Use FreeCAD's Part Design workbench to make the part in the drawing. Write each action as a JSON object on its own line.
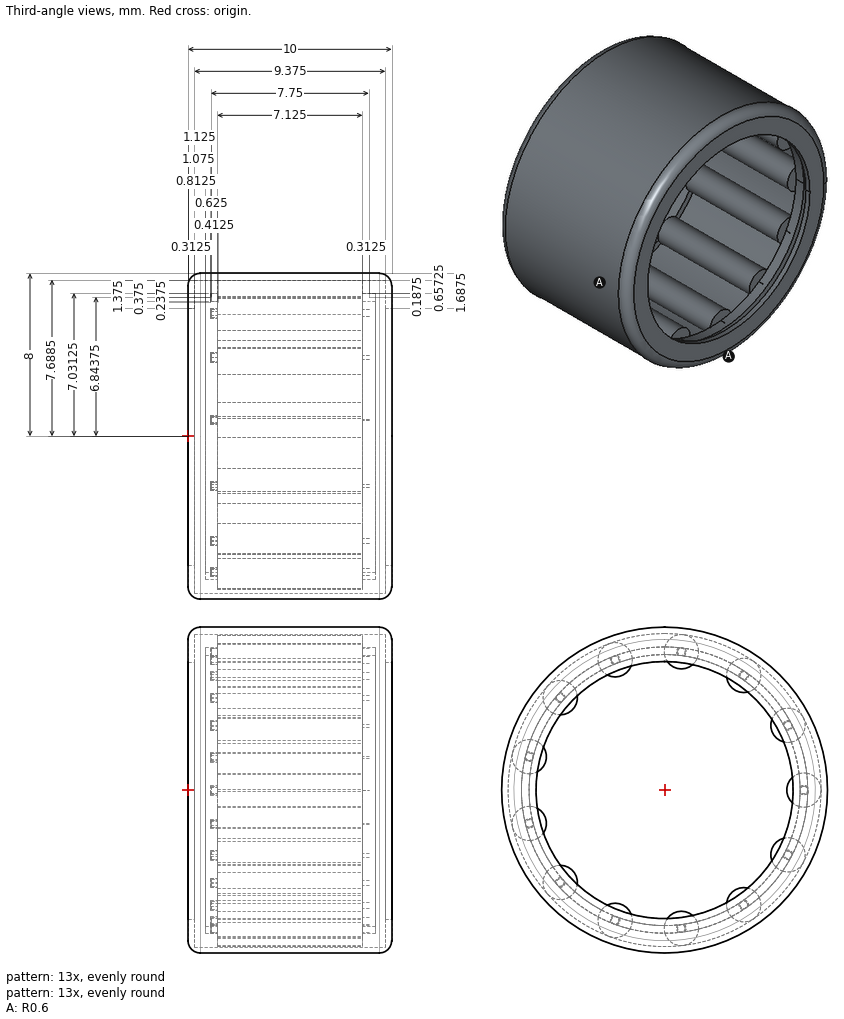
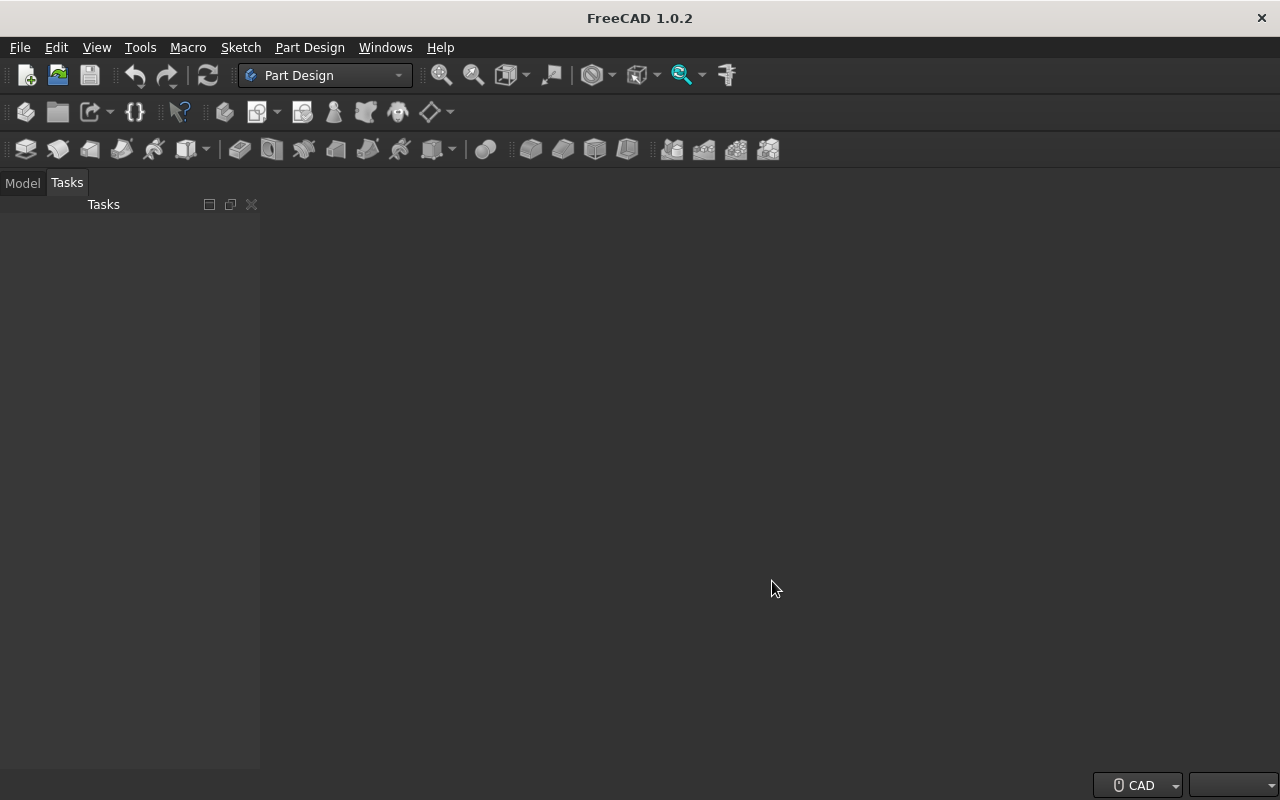
{"action": "left_click", "coordinate": [26, 76]}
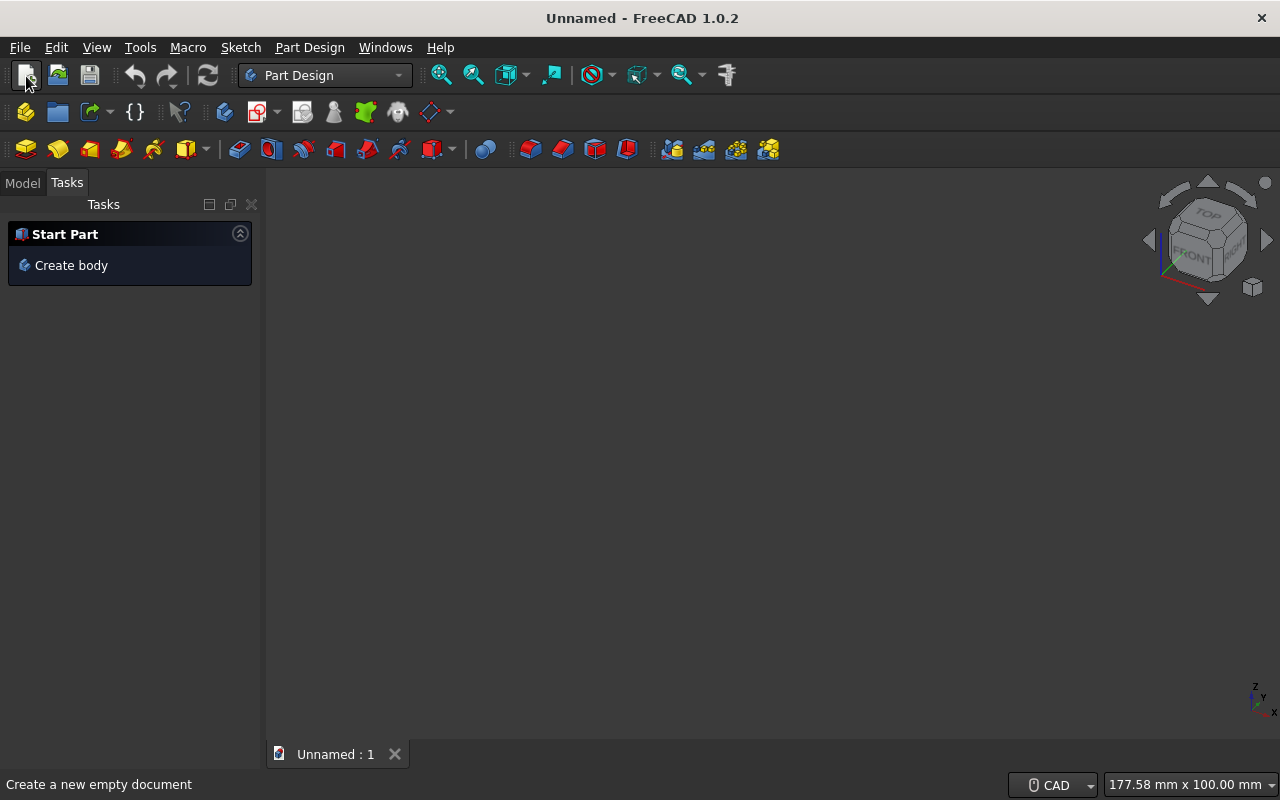
{"action": "left_click", "coordinate": [258, 112]}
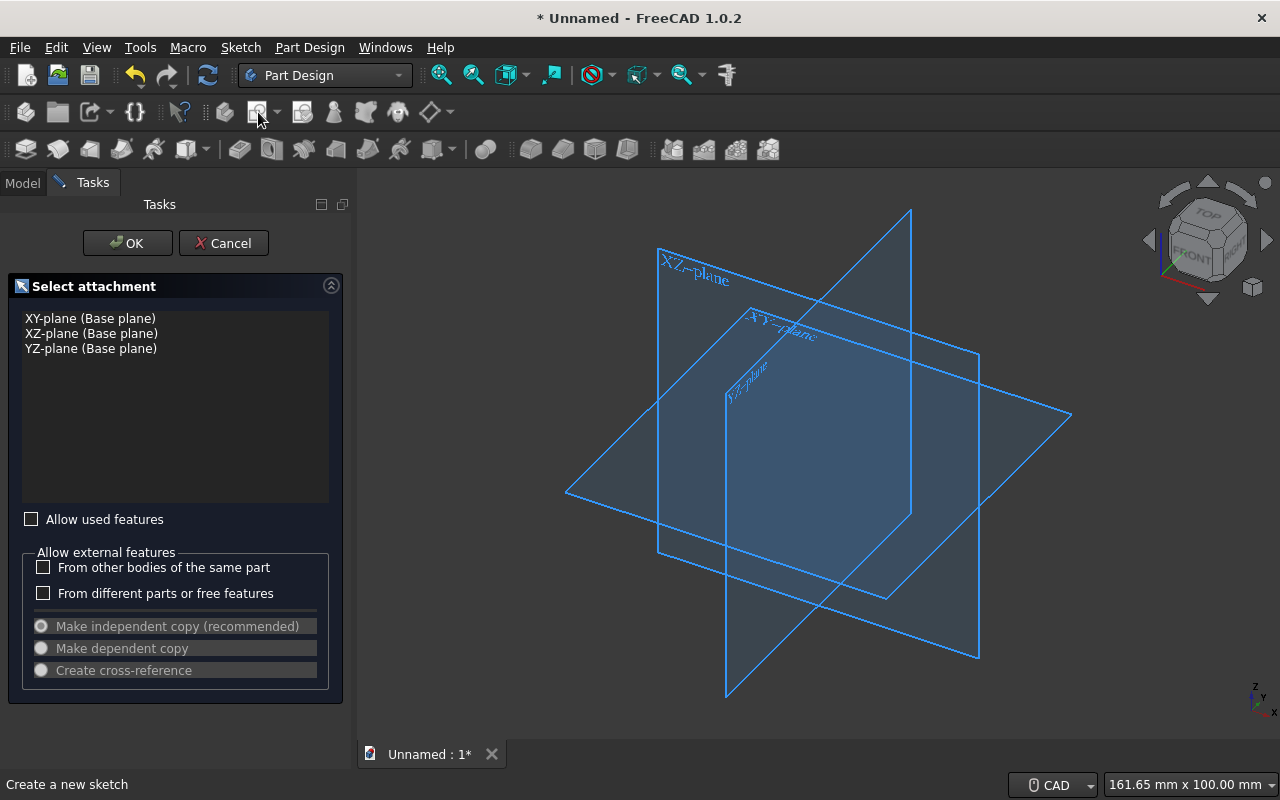
{"action": "left_click", "coordinate": [82, 318]}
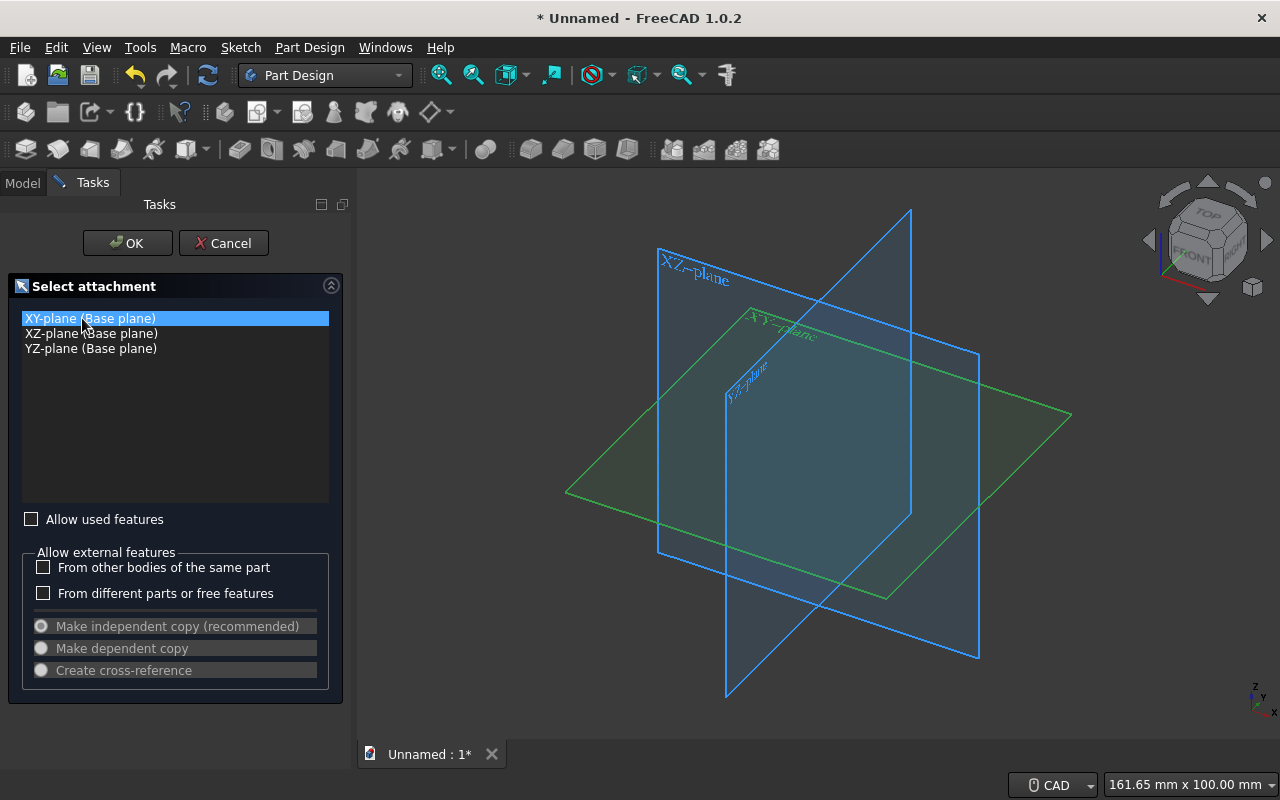
{"action": "left_click", "coordinate": [128, 243]}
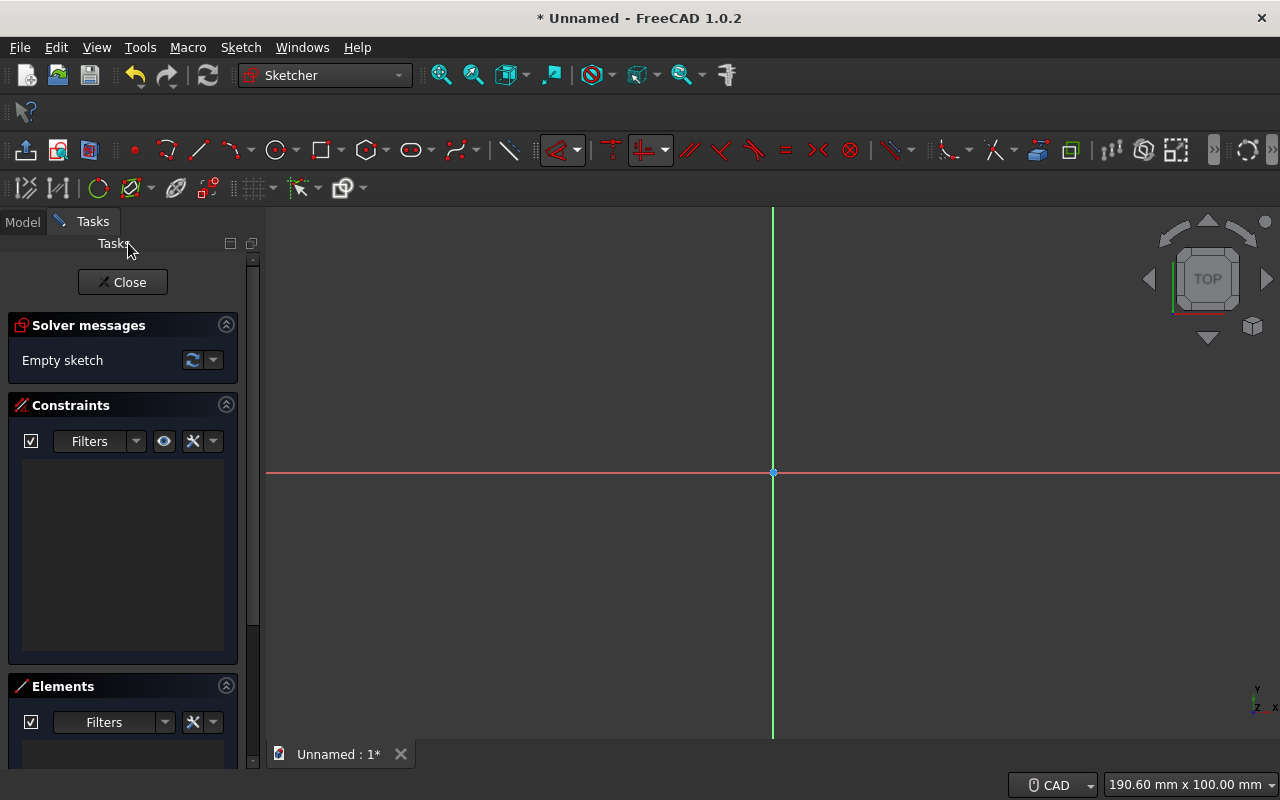
{"action": "scroll", "coordinate": [783, 435], "scroll_direction": "up", "scroll_amount": 15}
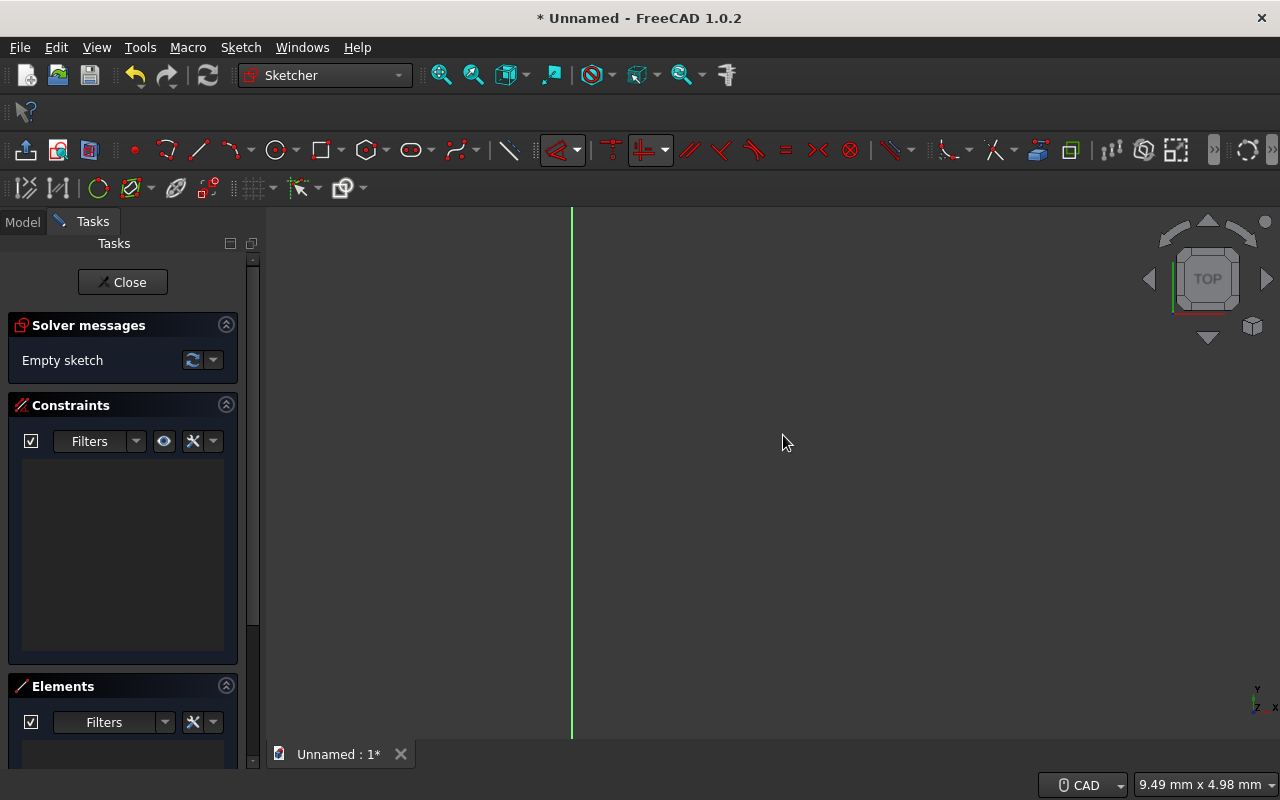
{"action": "scroll", "coordinate": [691, 457], "scroll_direction": "up", "scroll_amount": 11}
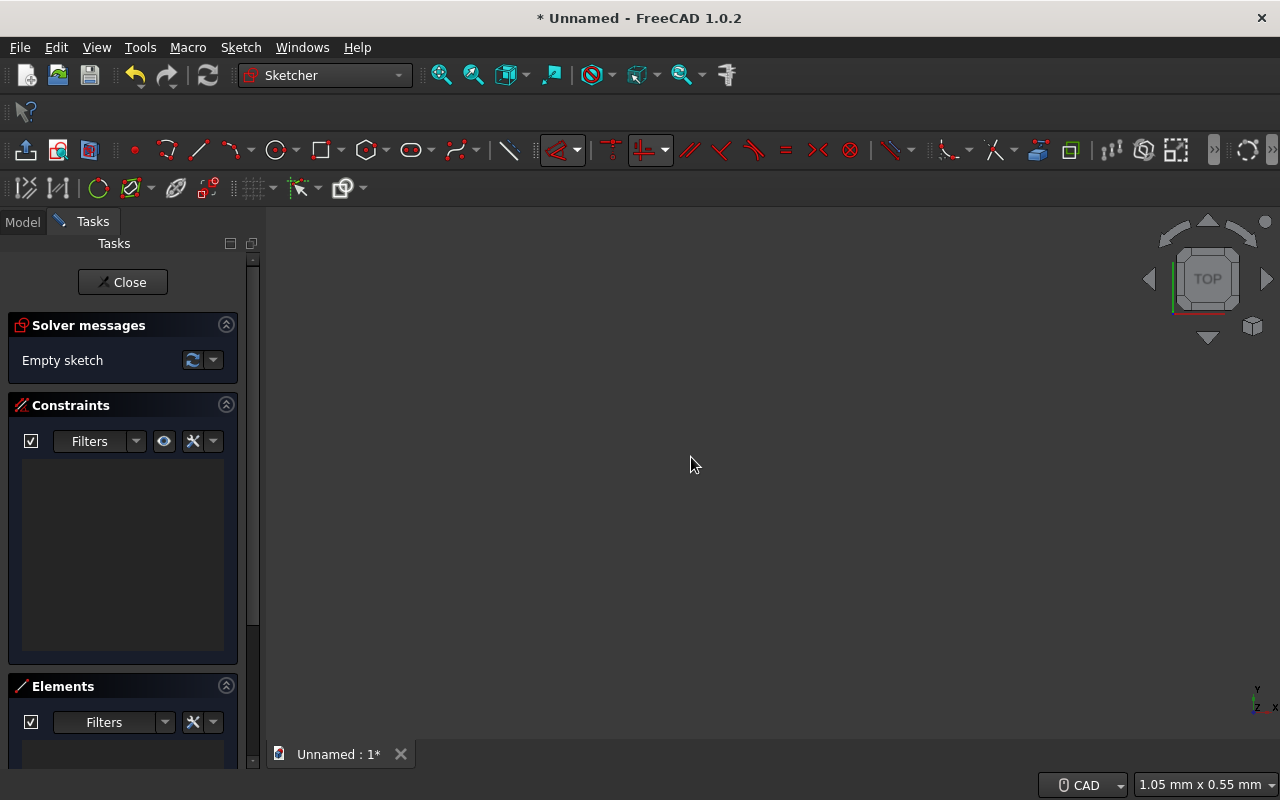
{"action": "left_click", "coordinate": [322, 150]}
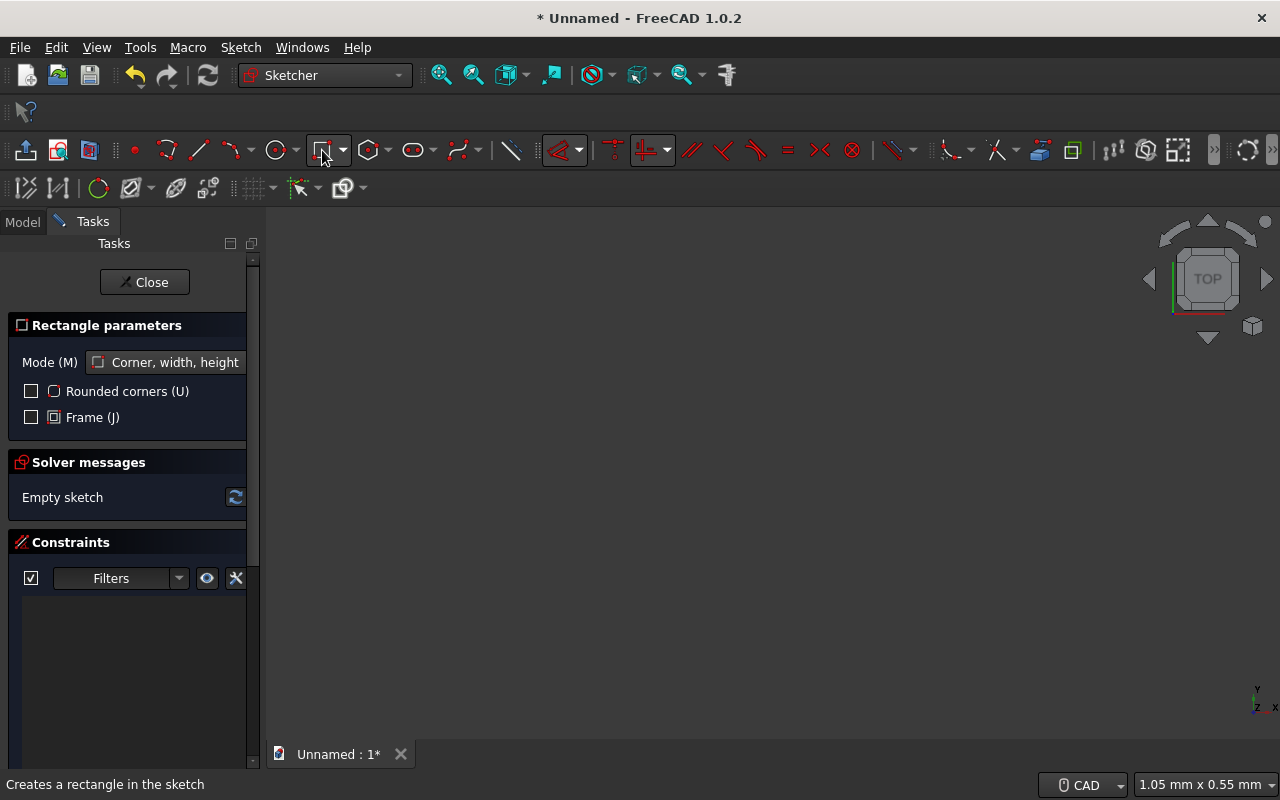
{"action": "left_click", "coordinate": [401, 288]}
{"action": "left_click", "coordinate": [1004, 650]}
{"action": "key", "text": "Escape"}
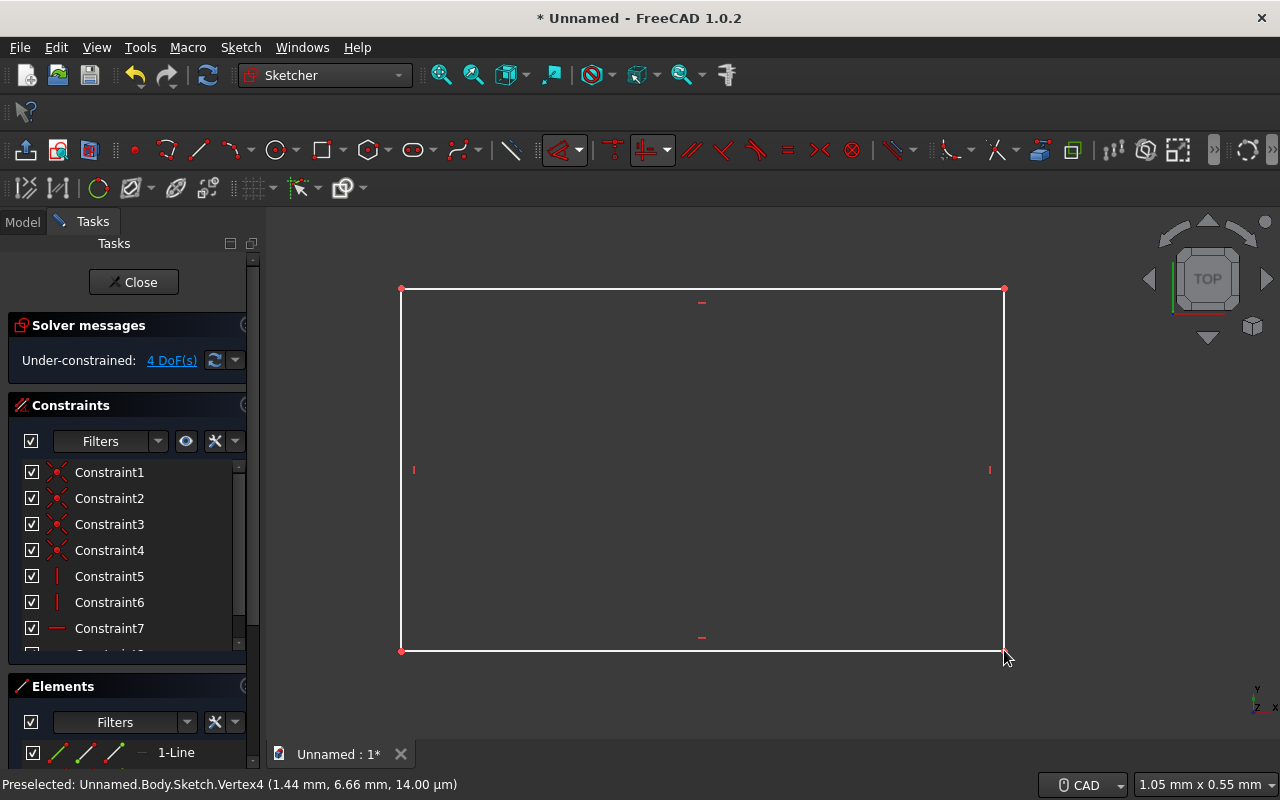
{"action": "left_click", "coordinate": [558, 150]}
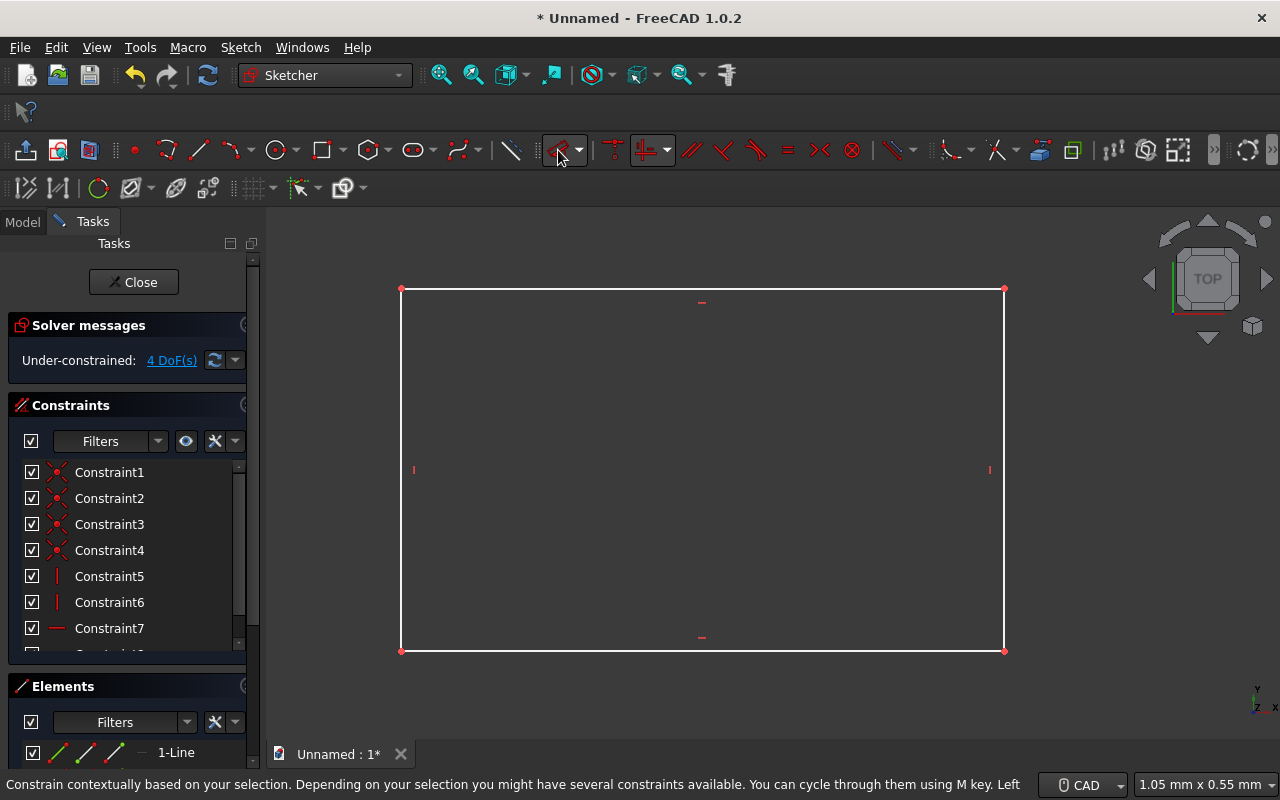
{"action": "left_click", "coordinate": [401, 398]}
{"action": "left_click", "coordinate": [367, 470]}